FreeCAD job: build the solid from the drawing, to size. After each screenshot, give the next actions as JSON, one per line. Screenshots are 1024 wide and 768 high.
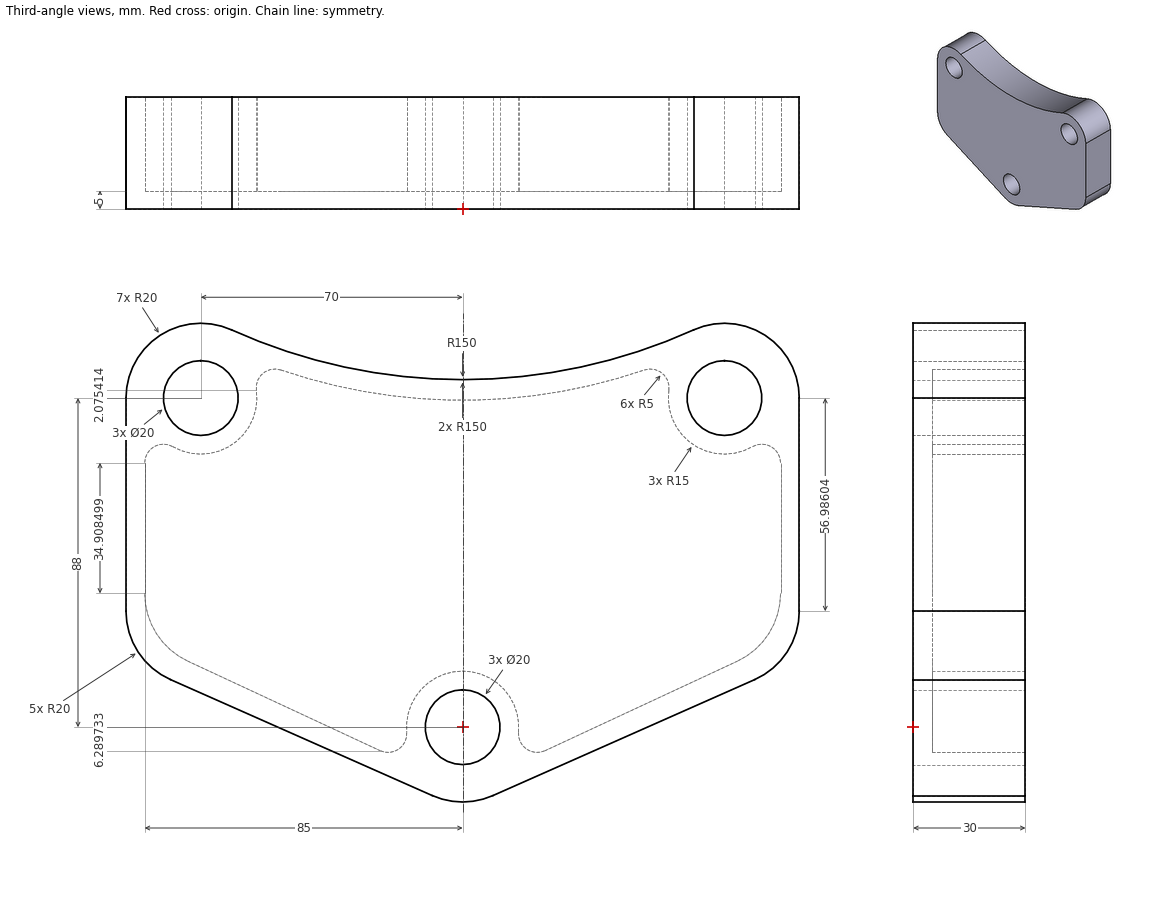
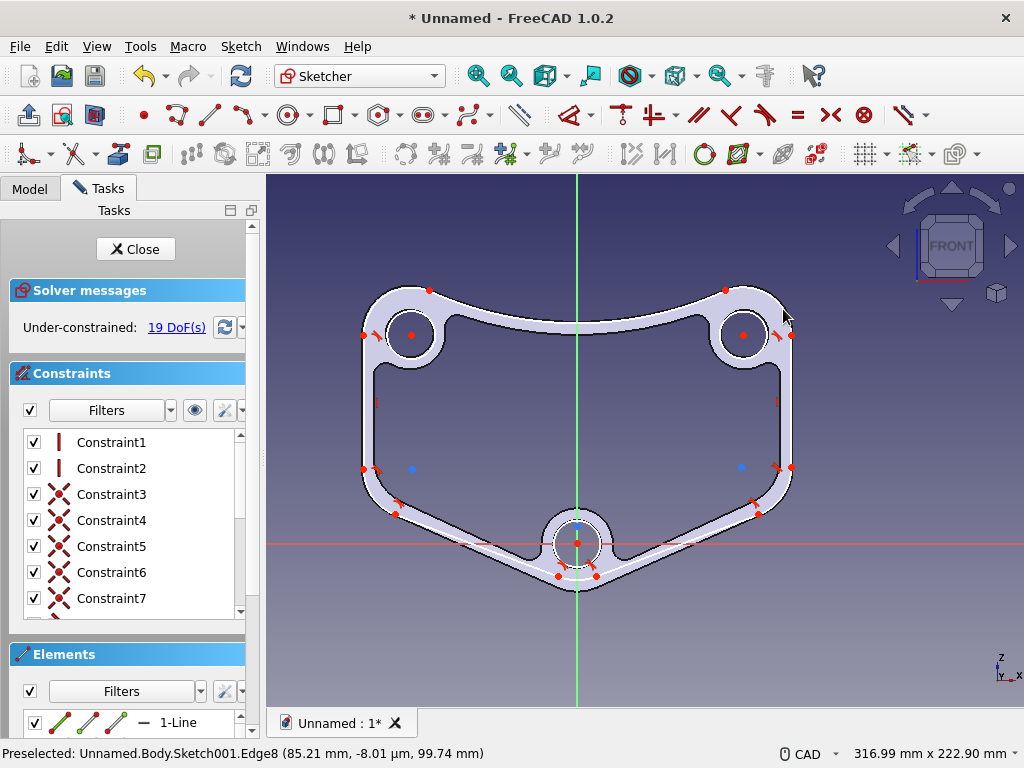
{"action": "left_click", "coordinate": [783, 309]}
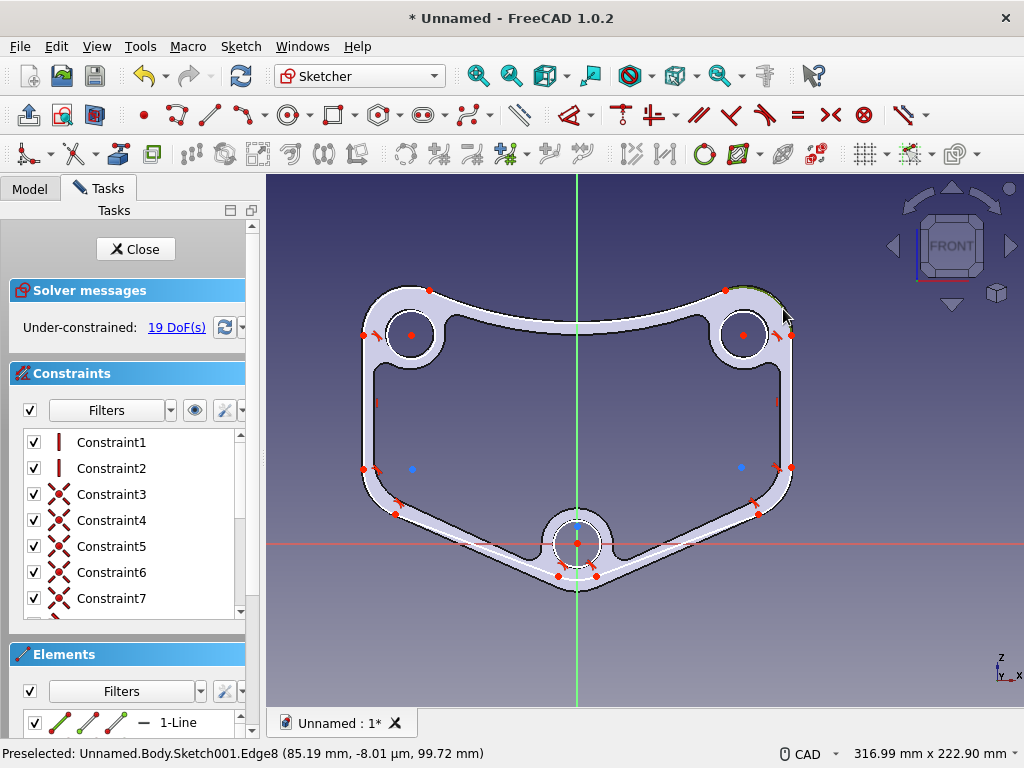
{"action": "left_click", "coordinate": [516, 318]}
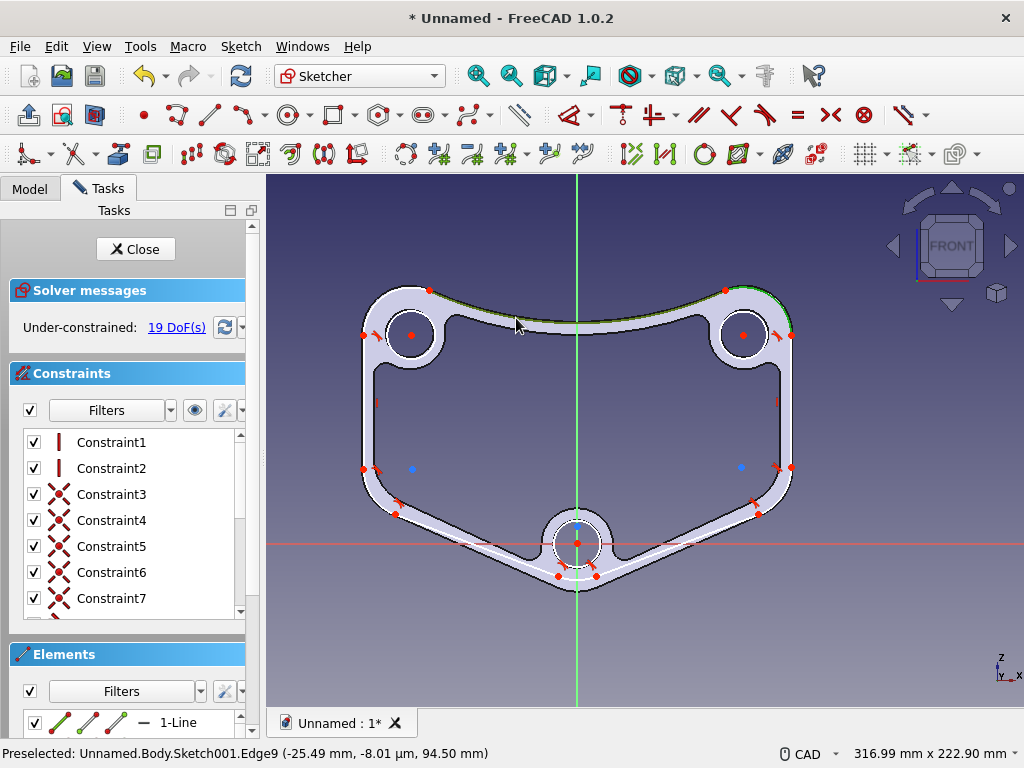
{"action": "left_click", "coordinate": [765, 116]}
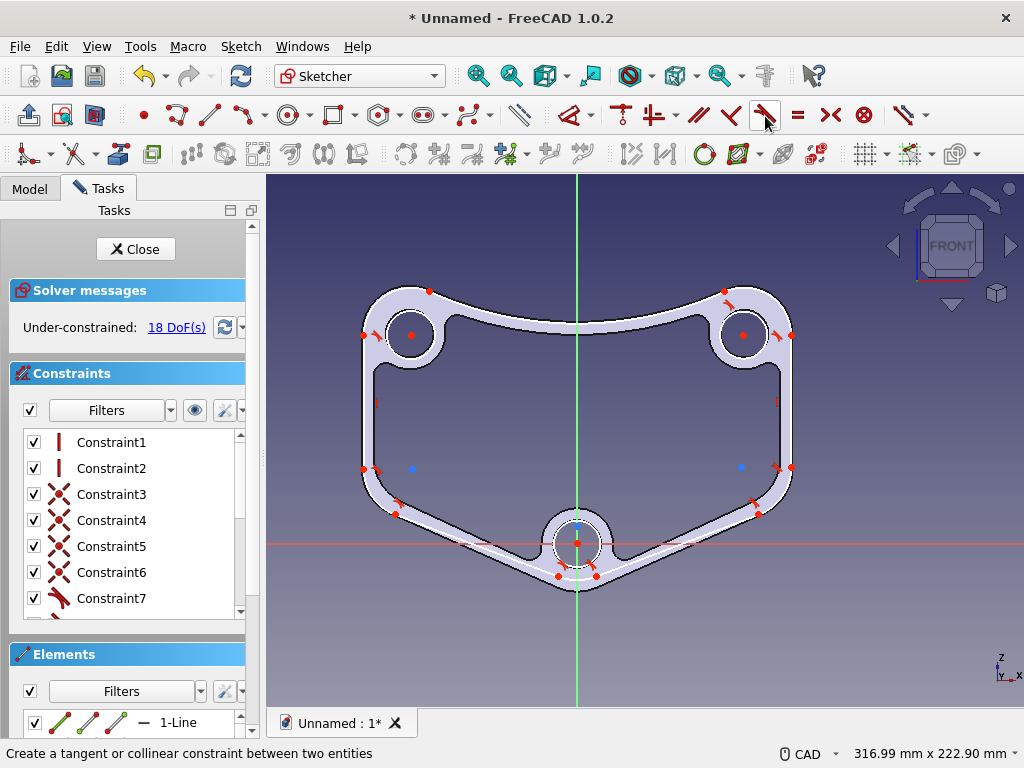
{"action": "left_click", "coordinate": [516, 318]}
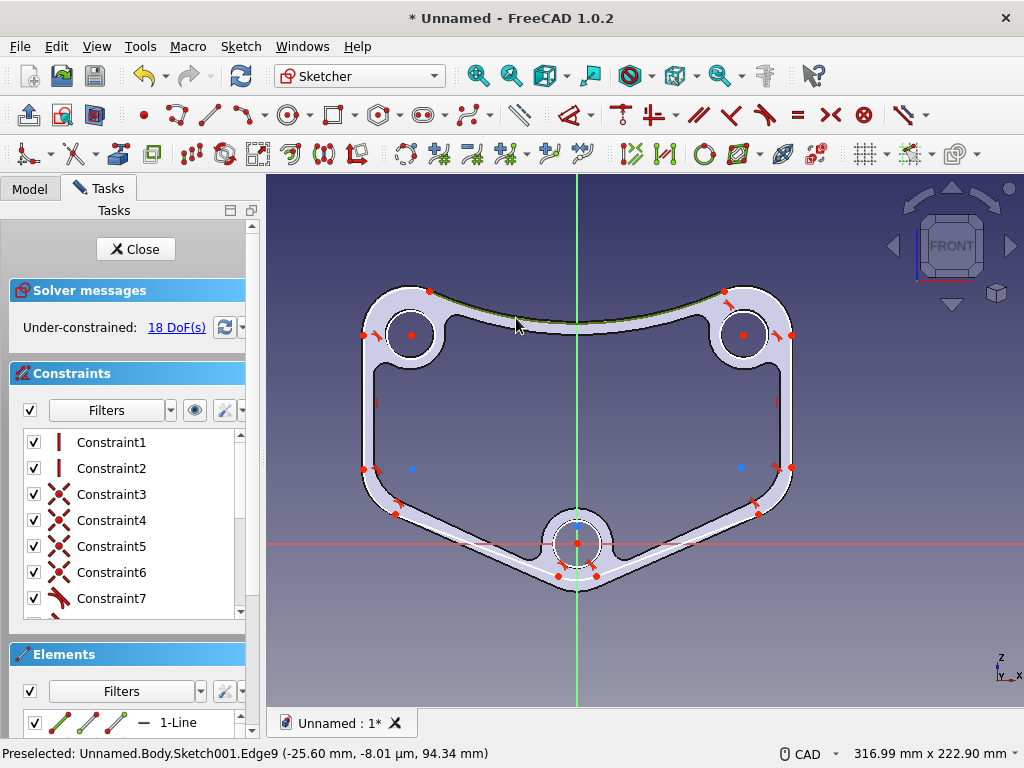
{"action": "left_click", "coordinate": [402, 289]}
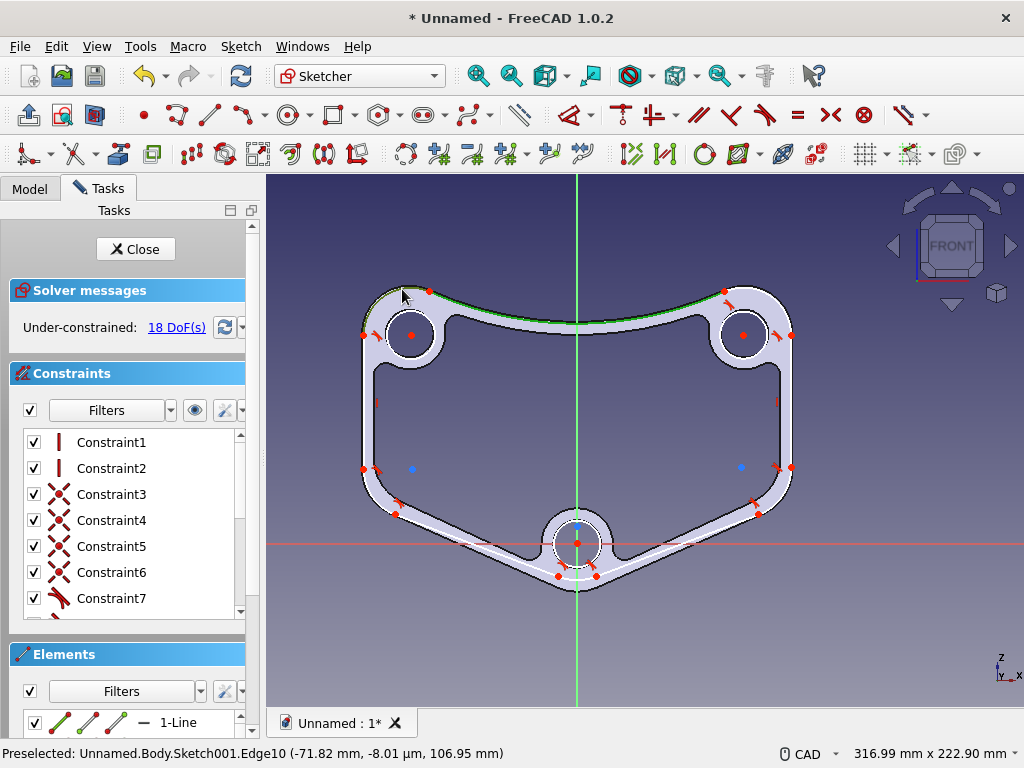
{"action": "left_click", "coordinate": [765, 116]}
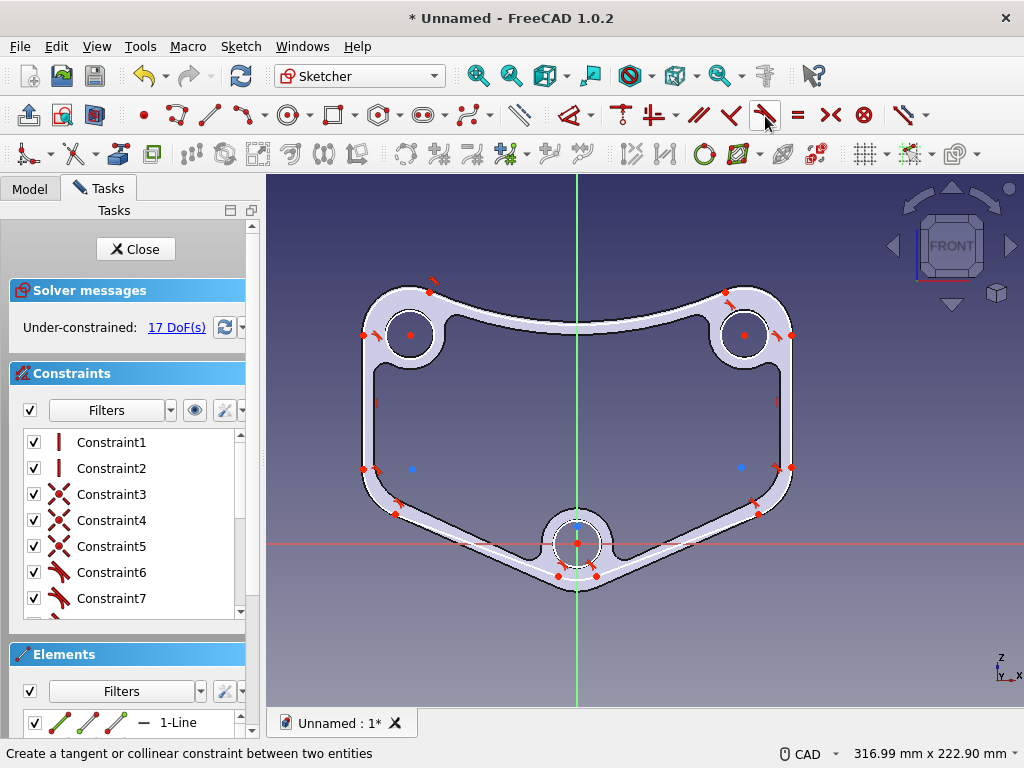
{"action": "left_click", "coordinate": [594, 528]}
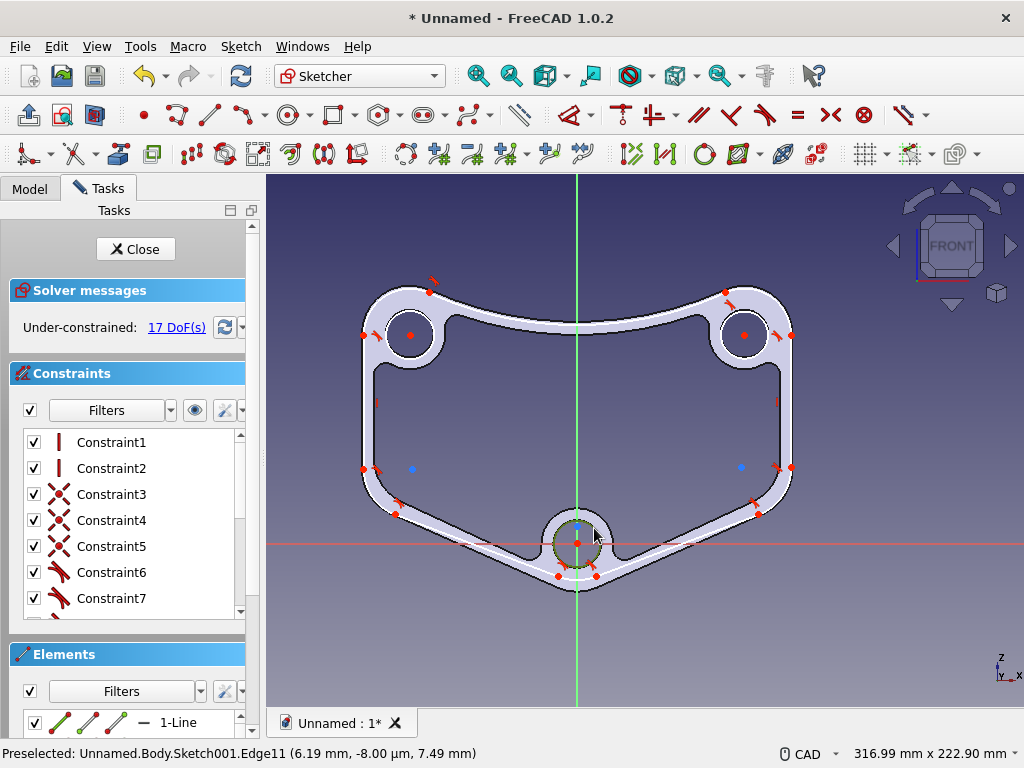
{"action": "left_click", "coordinate": [577, 580]}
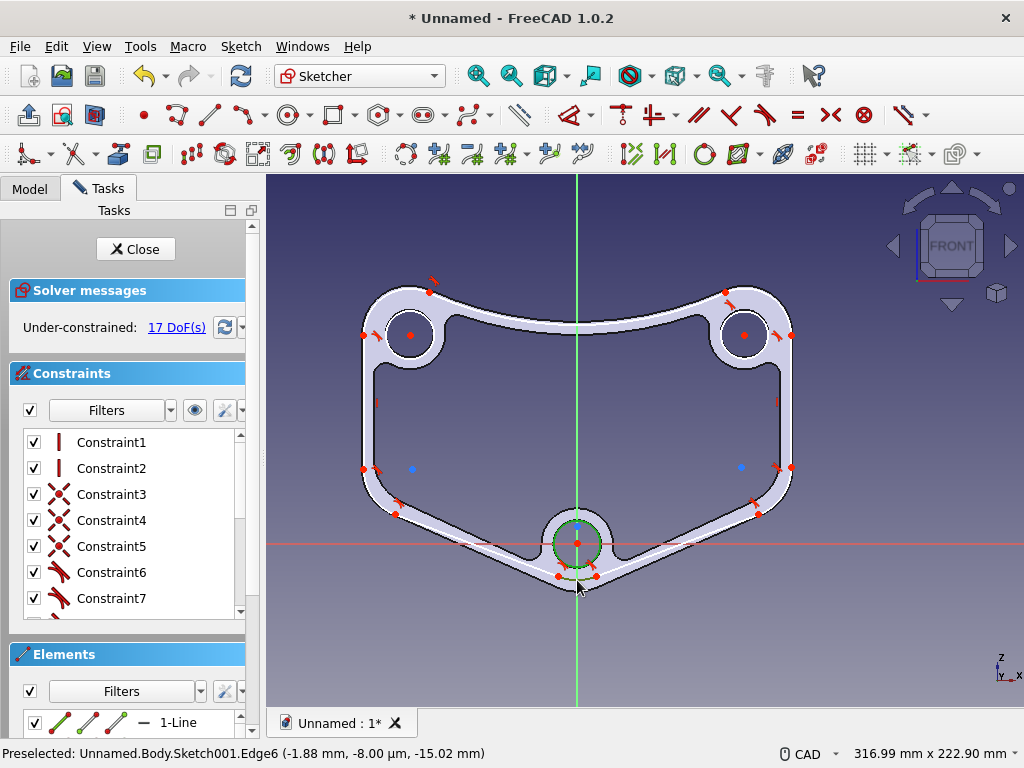
{"action": "left_click", "coordinate": [621, 116]}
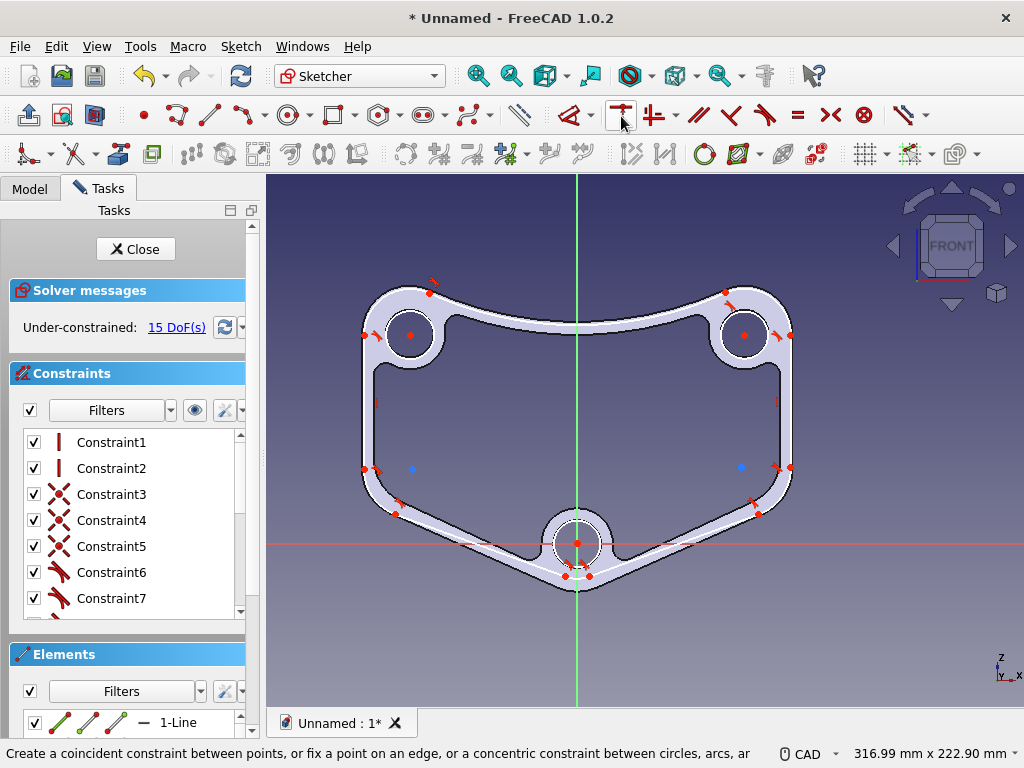
{"action": "left_click", "coordinate": [367, 487]}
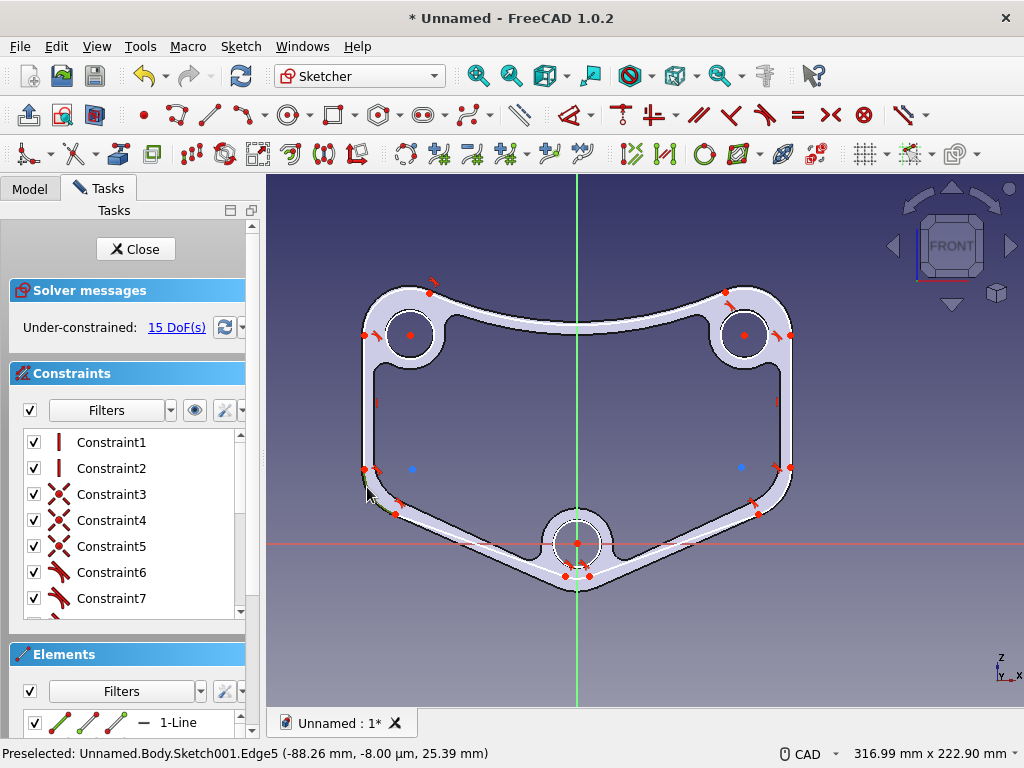
{"action": "left_click", "coordinate": [577, 579]}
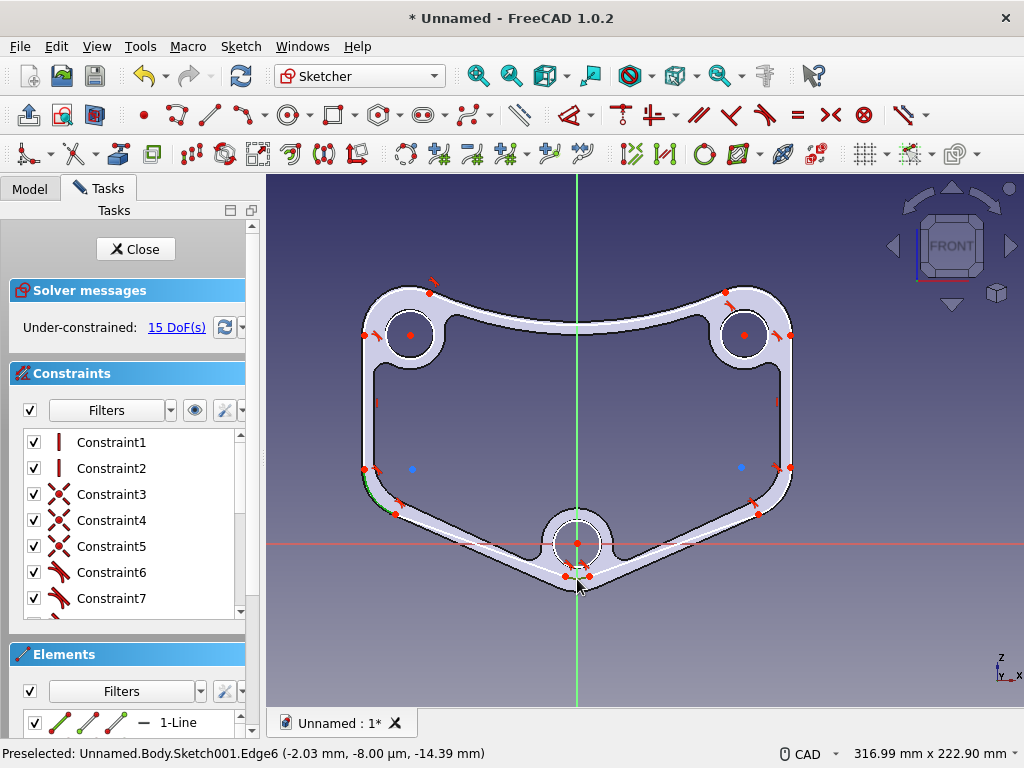
{"action": "left_click", "coordinate": [774, 505]}